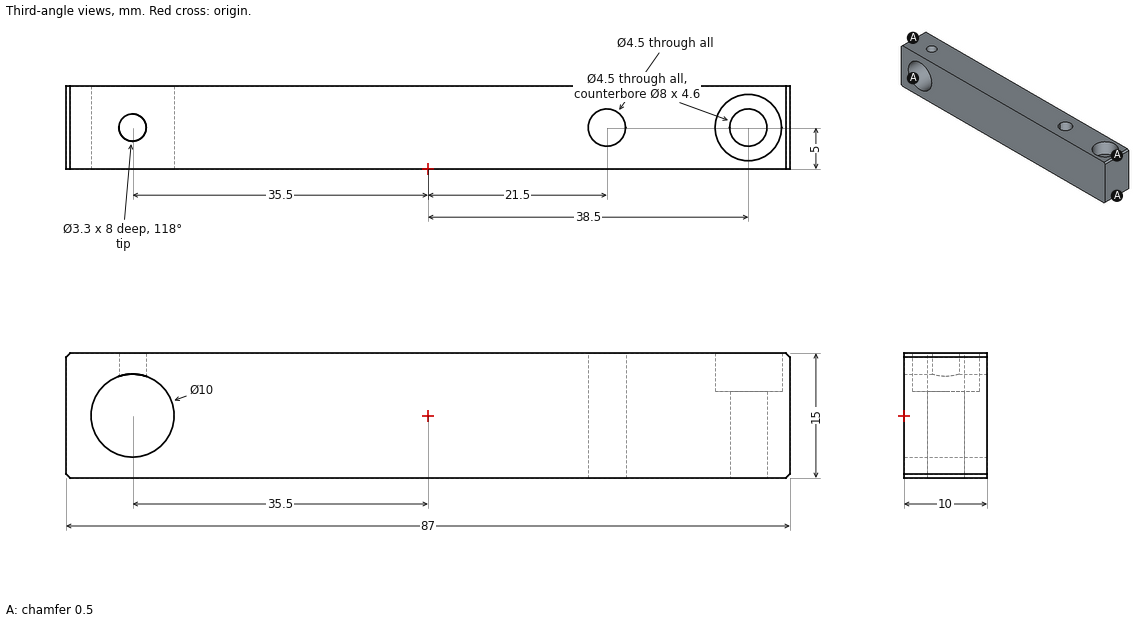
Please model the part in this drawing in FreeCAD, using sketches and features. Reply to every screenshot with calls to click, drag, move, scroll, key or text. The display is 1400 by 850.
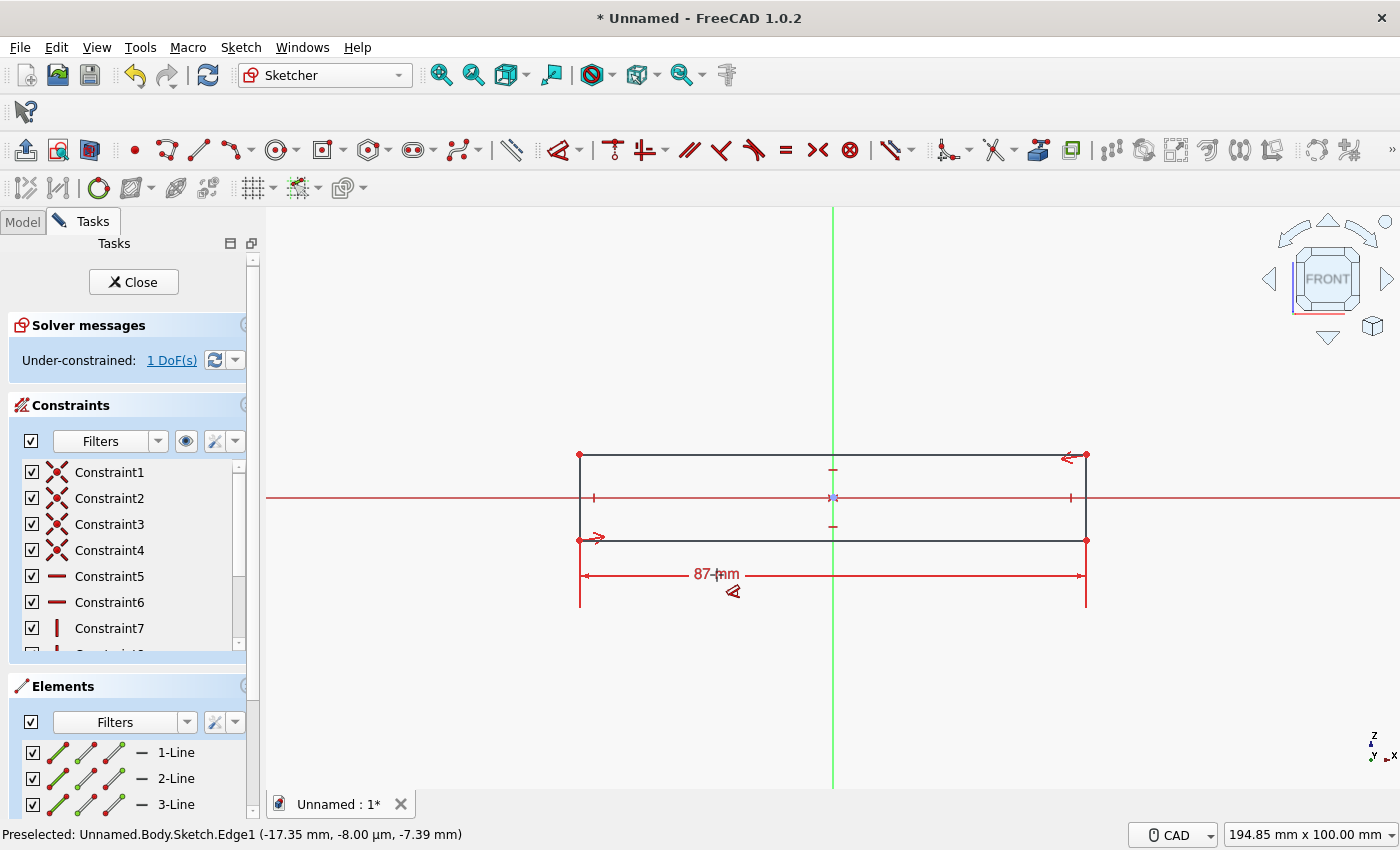
click(1086, 515)
click(1120, 478)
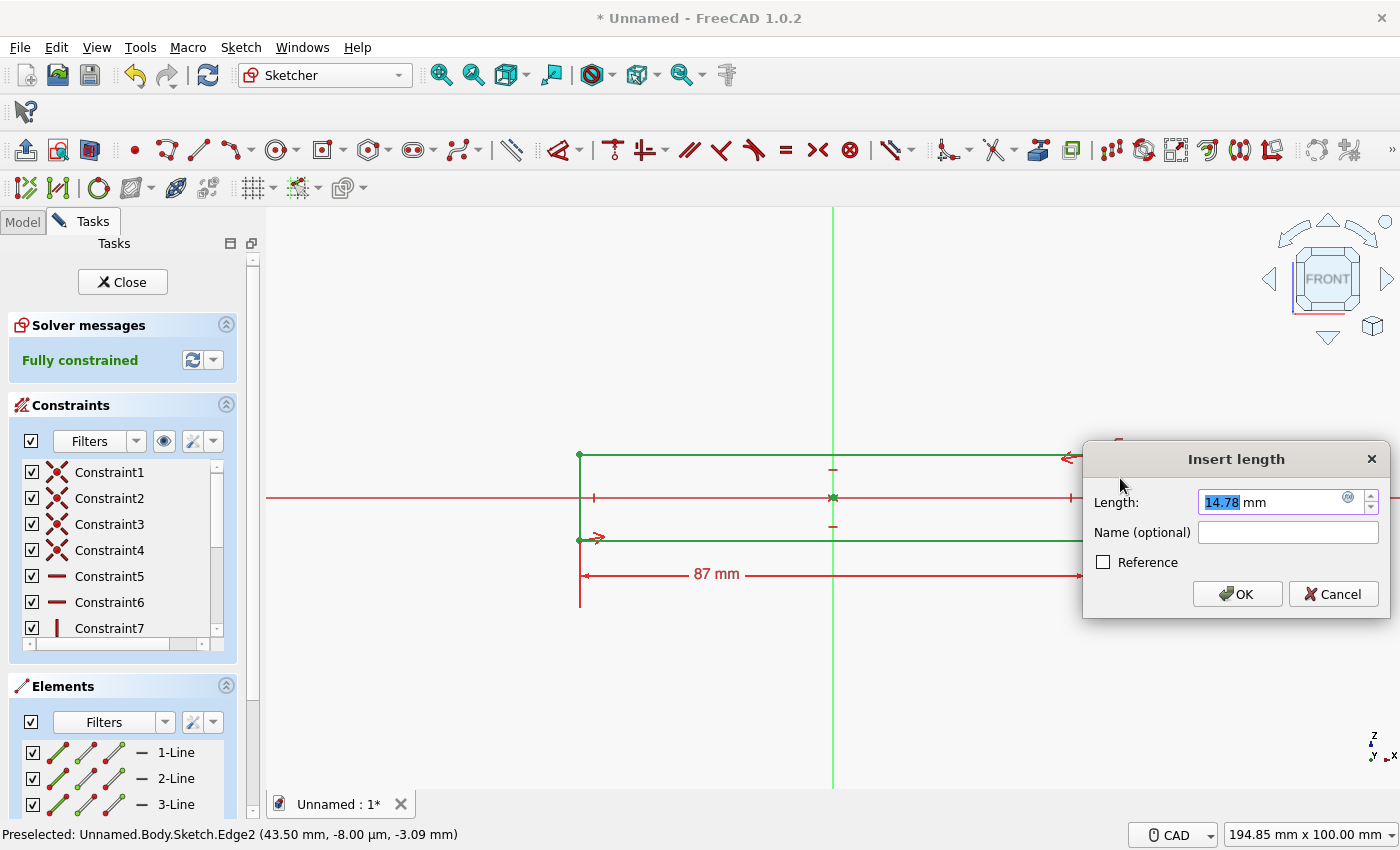
text(15)
key(Return)
key(Escape)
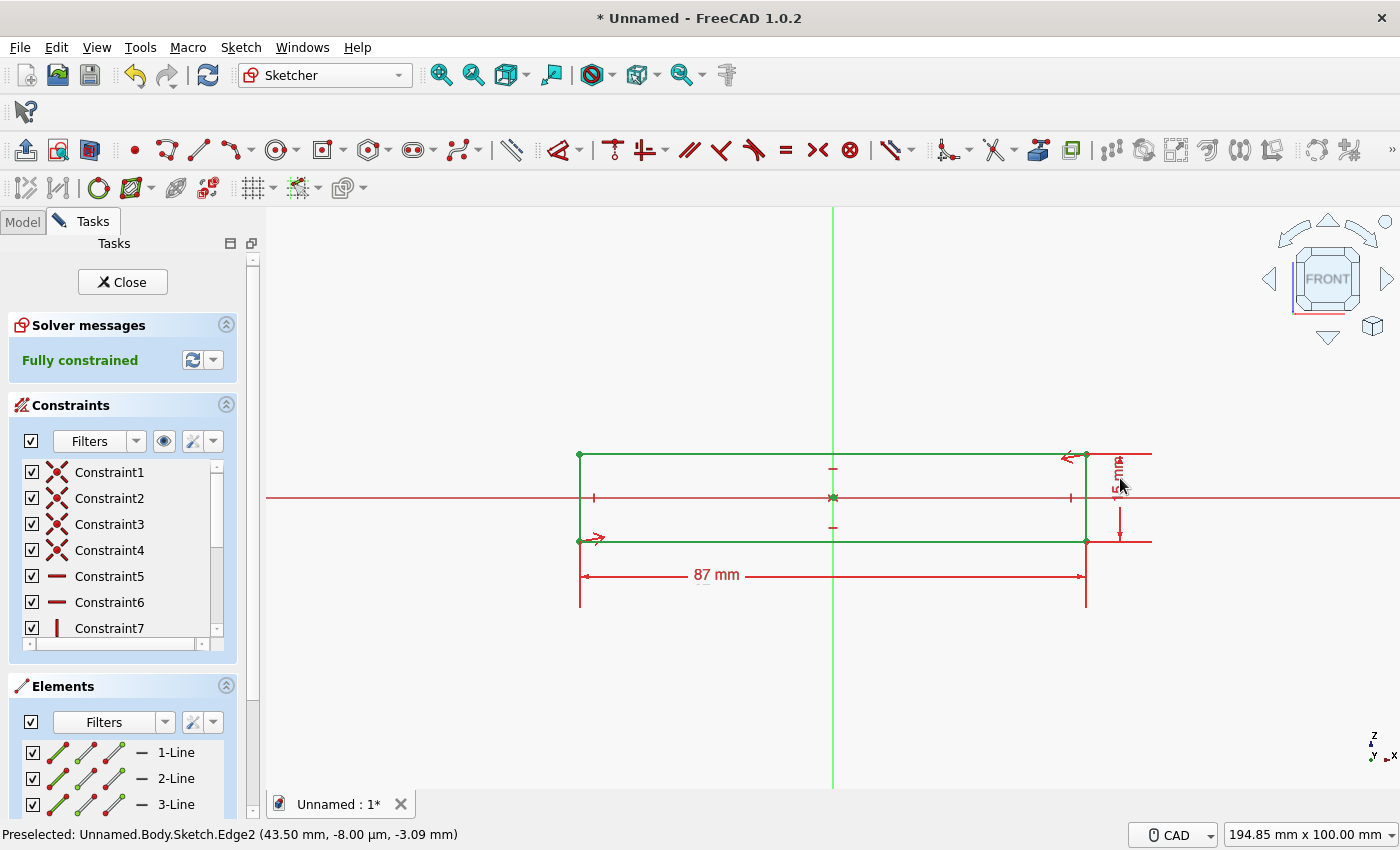
click(123, 282)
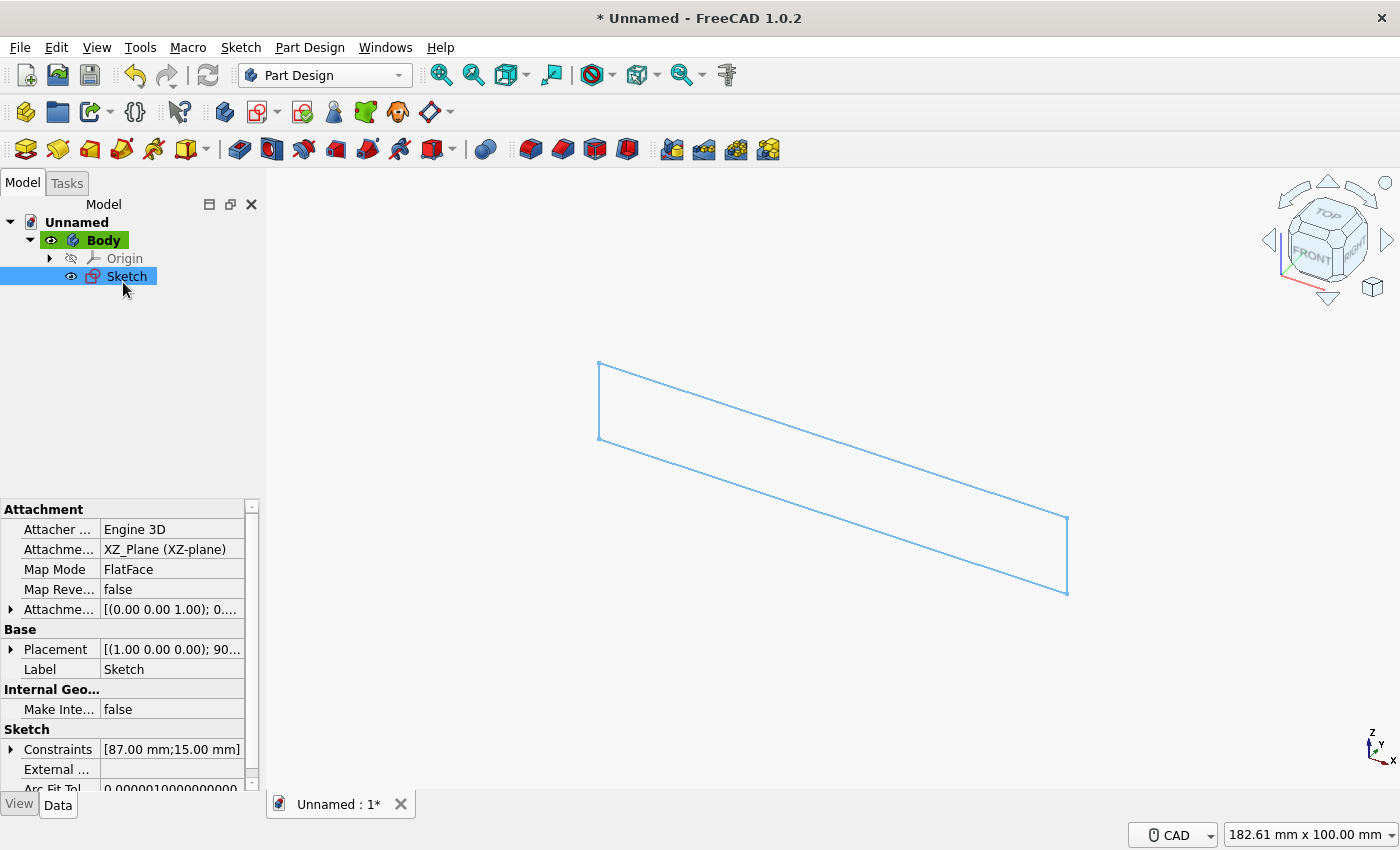
click(26, 150)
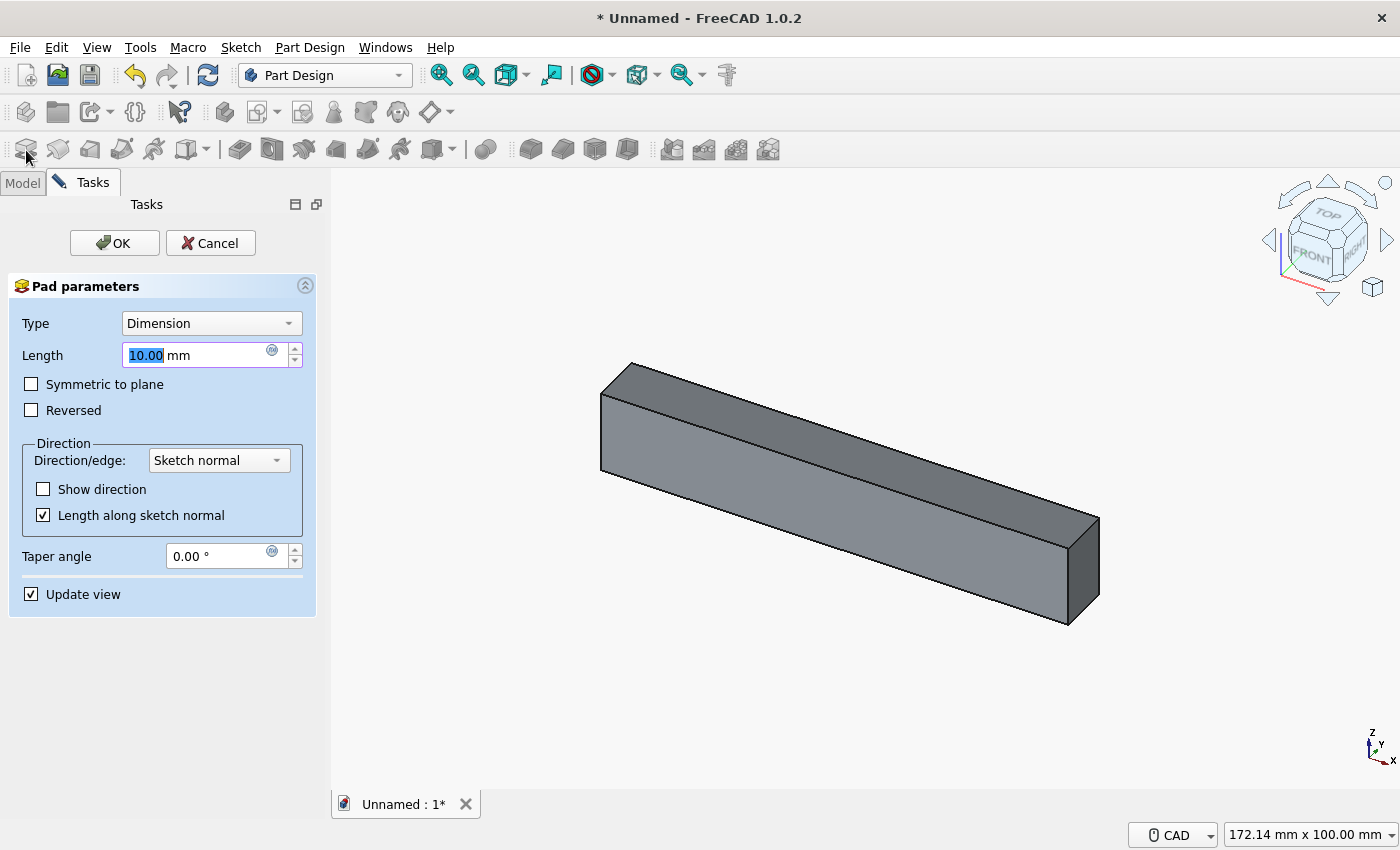
text(10)
key(Tab)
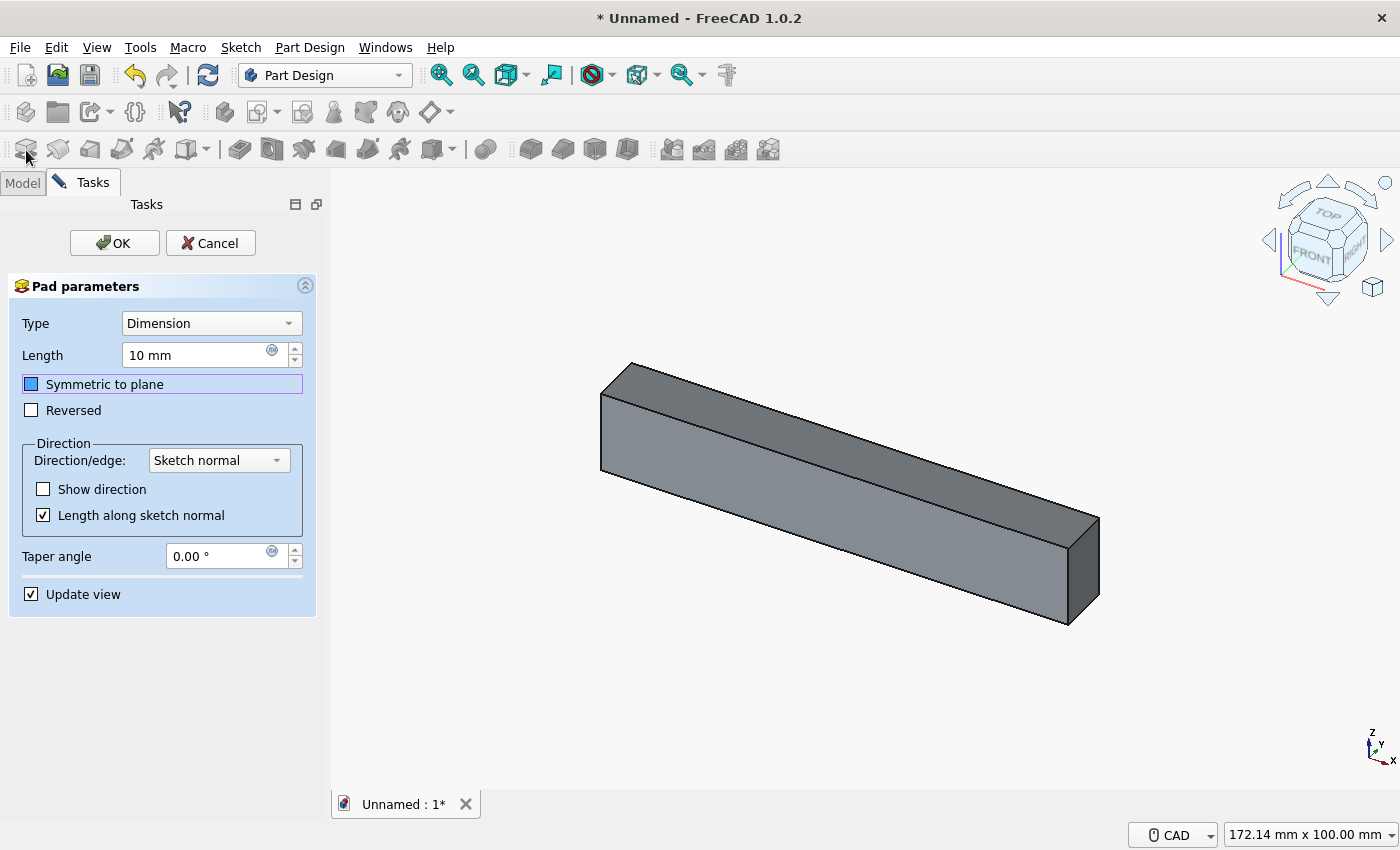
click(30, 410)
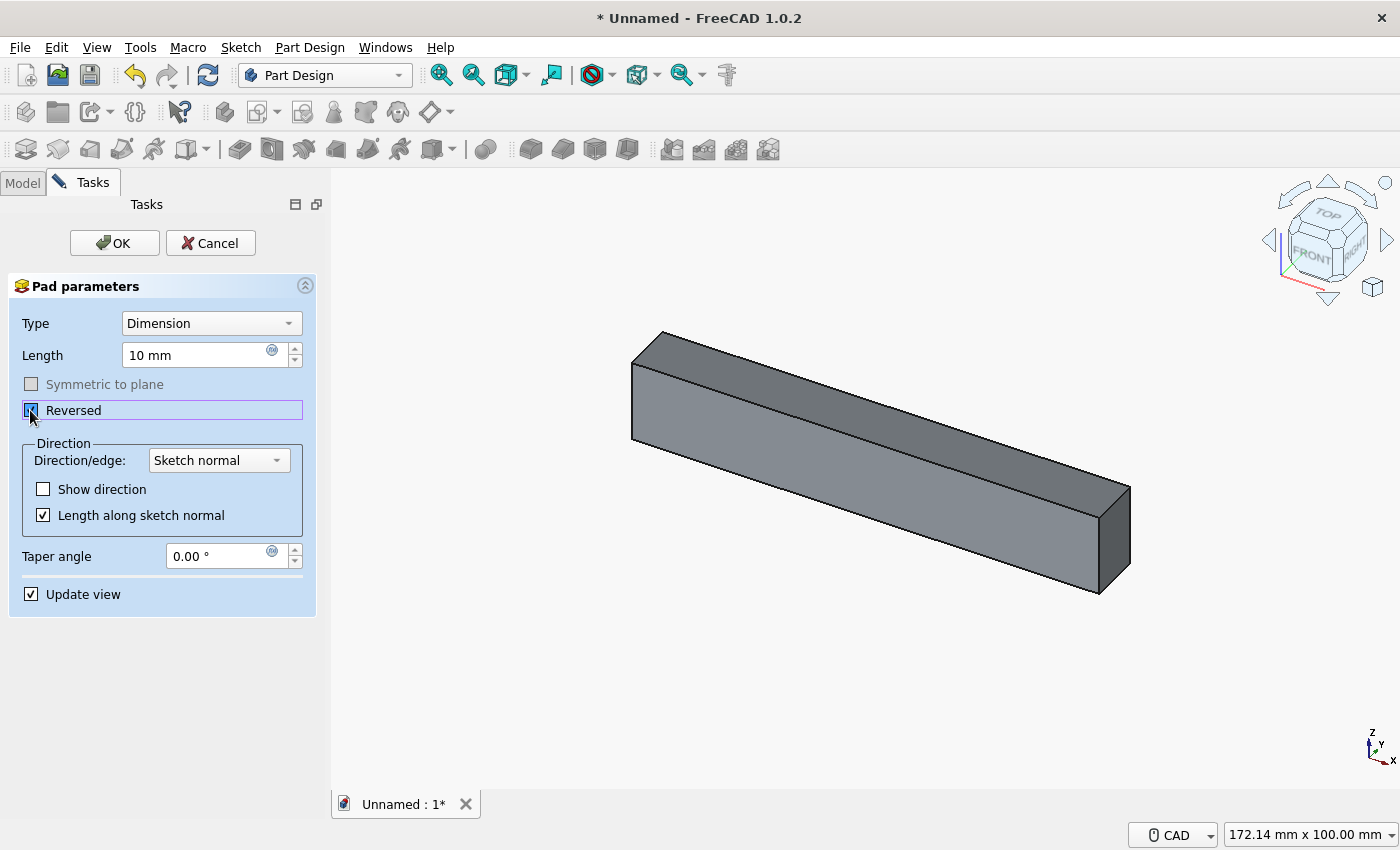
click(115, 243)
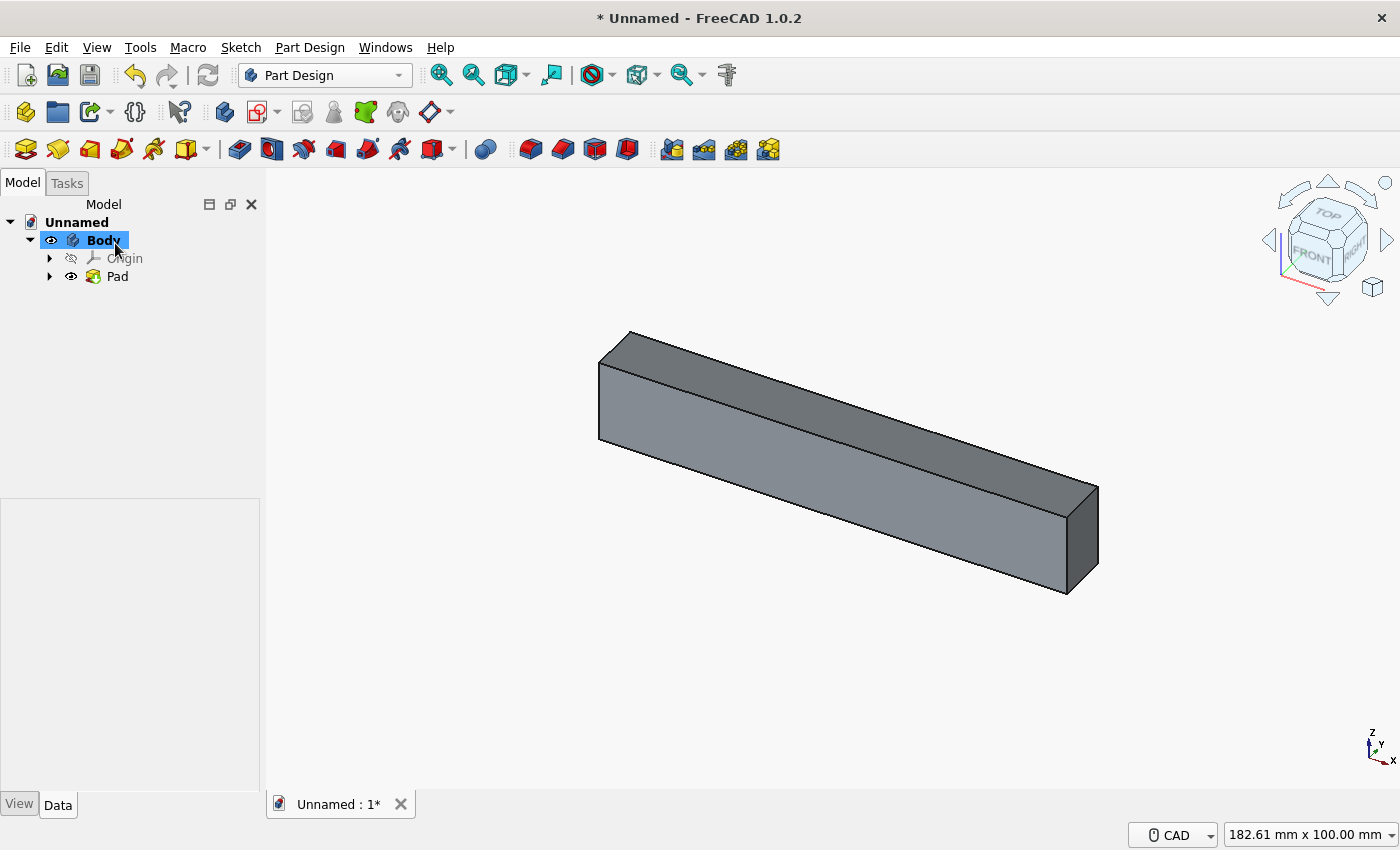
click(442, 76)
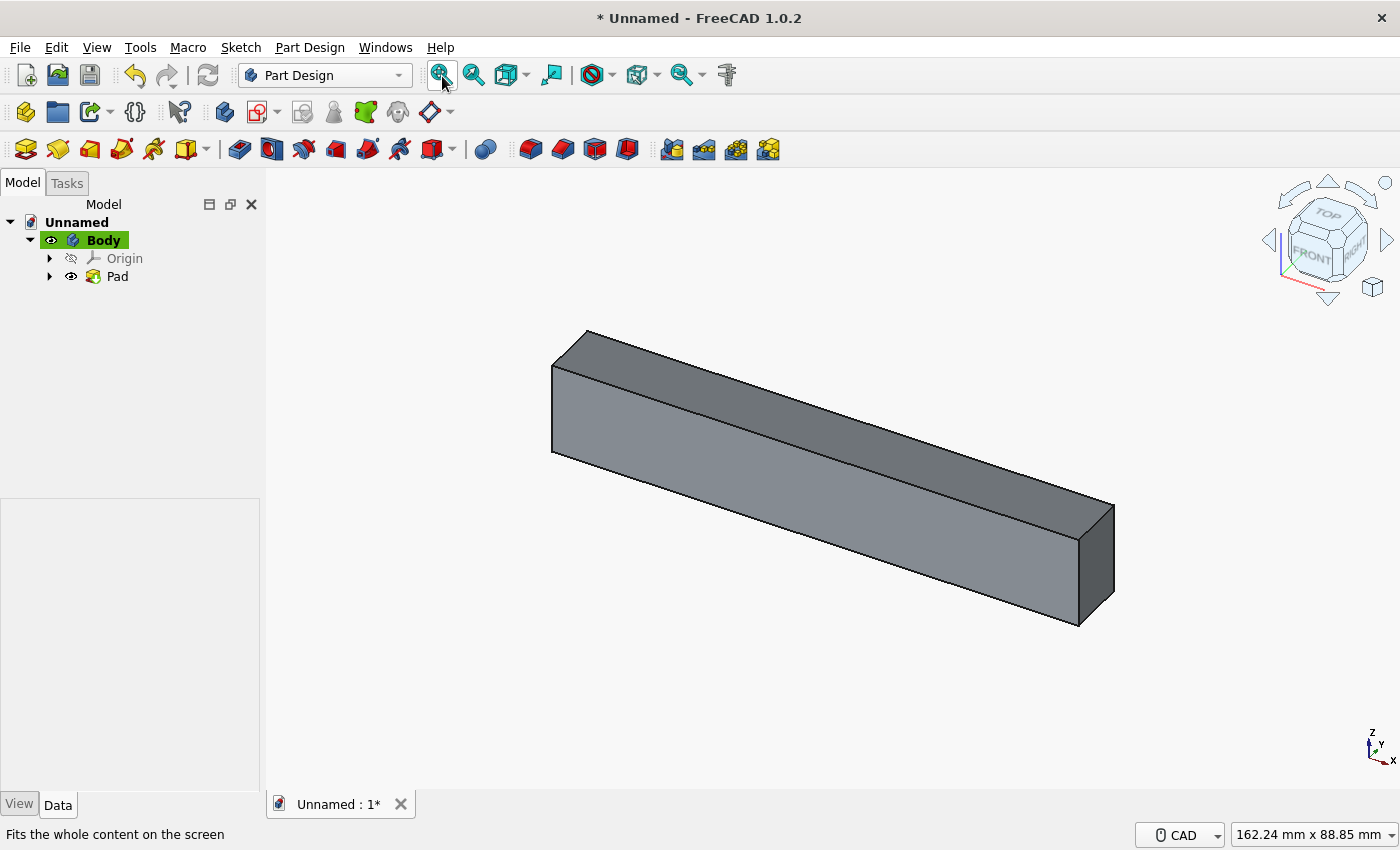
key(4)